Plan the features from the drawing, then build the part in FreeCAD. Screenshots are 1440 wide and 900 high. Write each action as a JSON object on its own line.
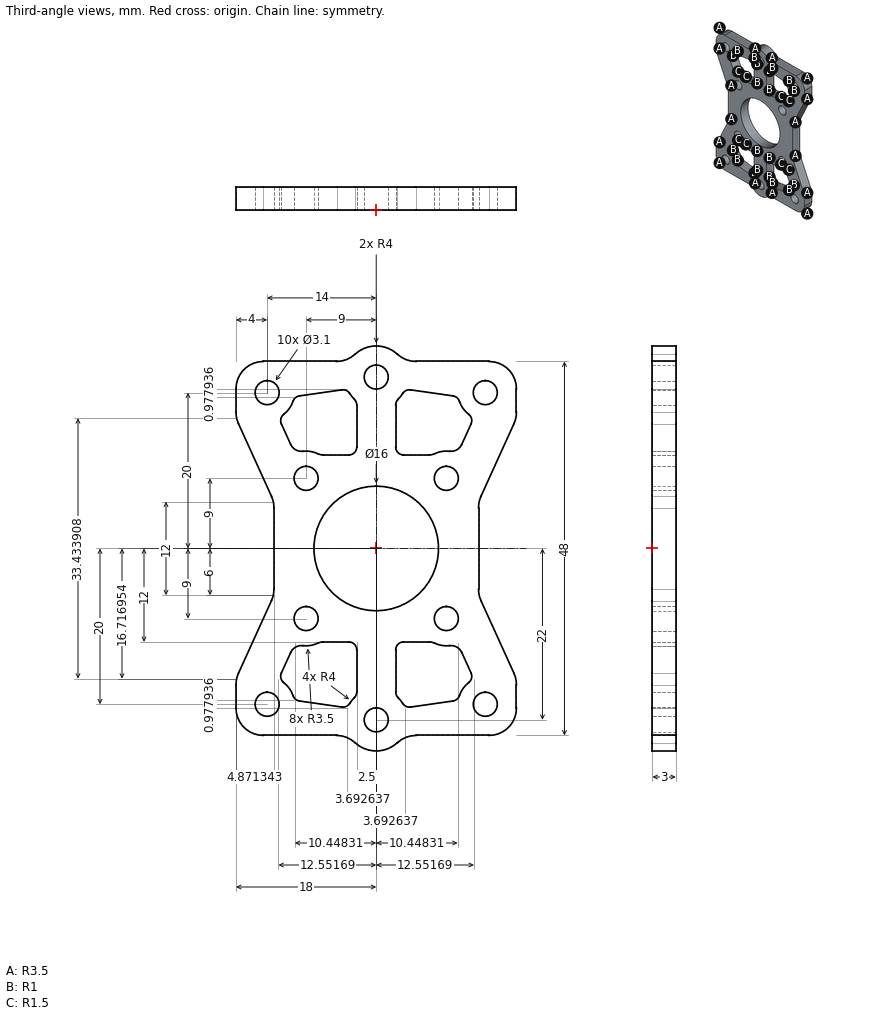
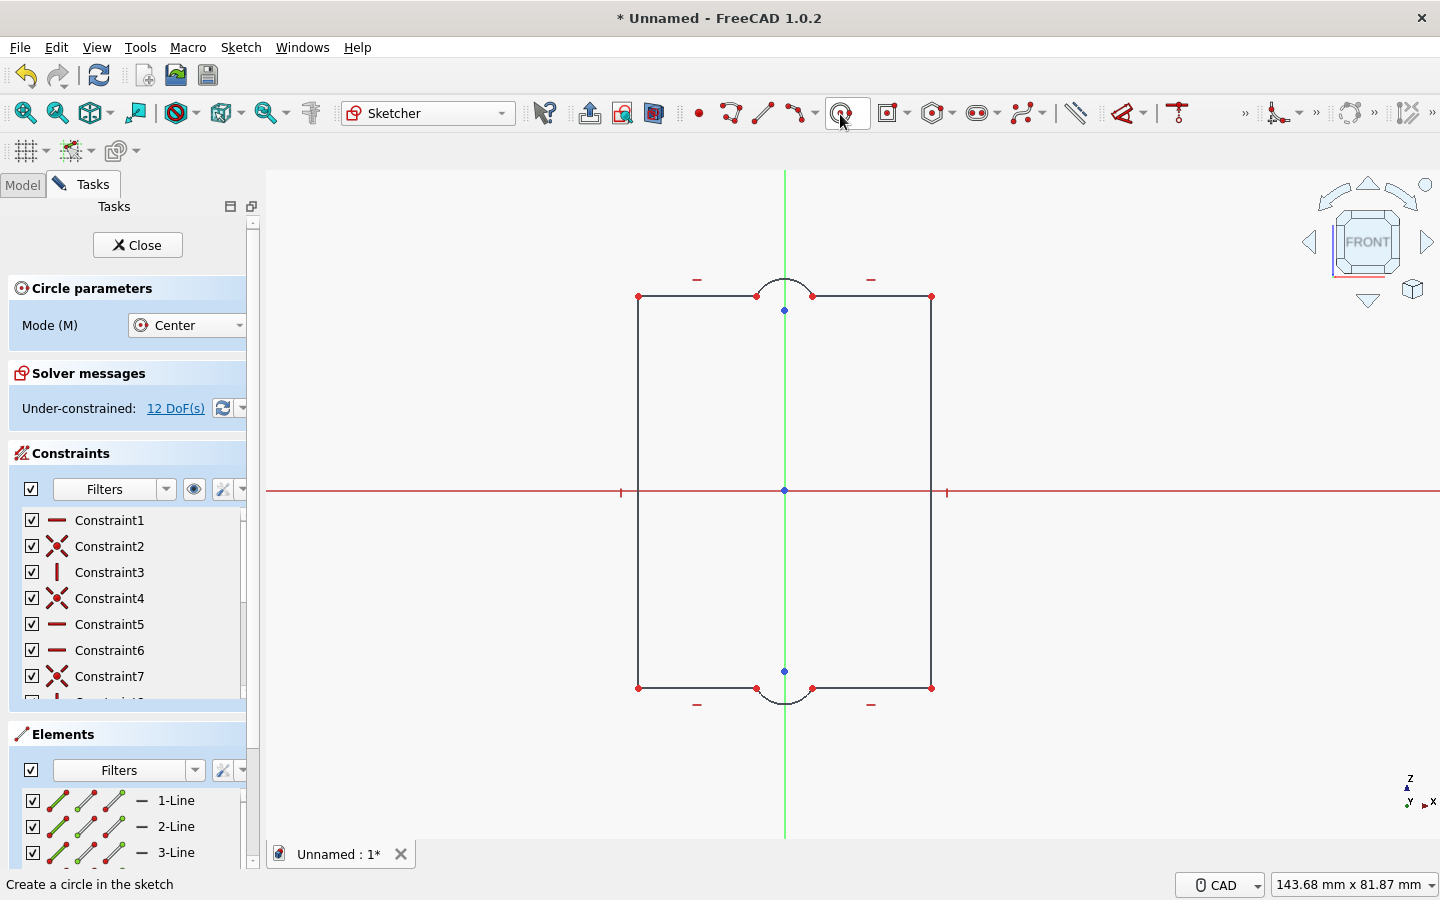
{"action": "scroll", "coordinate": [670, 327], "scroll_direction": "up", "scroll_amount": 3}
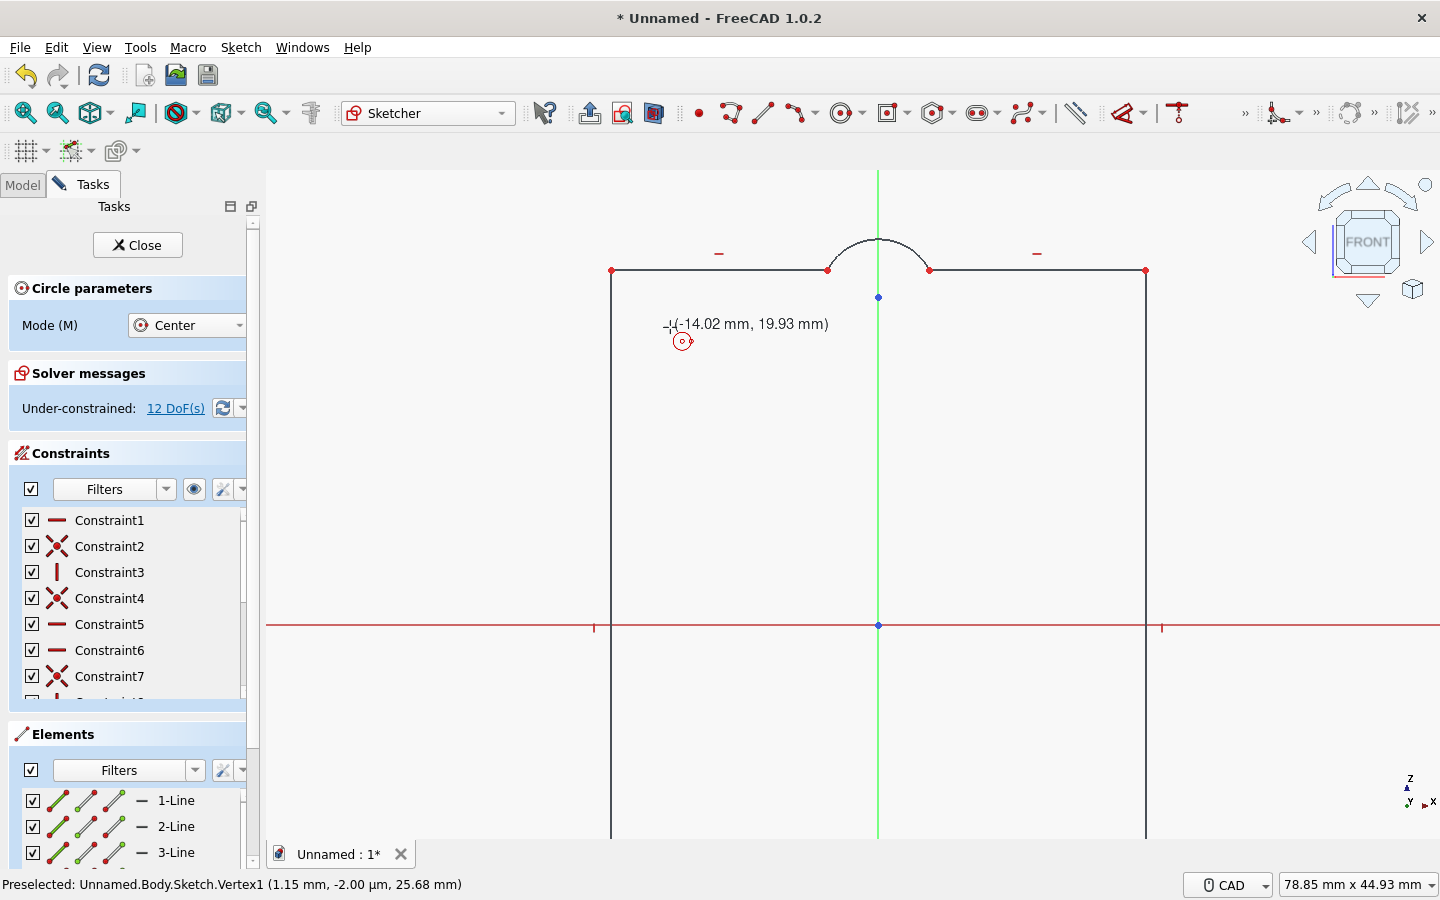
{"action": "left_click", "coordinate": [670, 328]}
{"action": "mouse_move", "coordinate": [686, 311]}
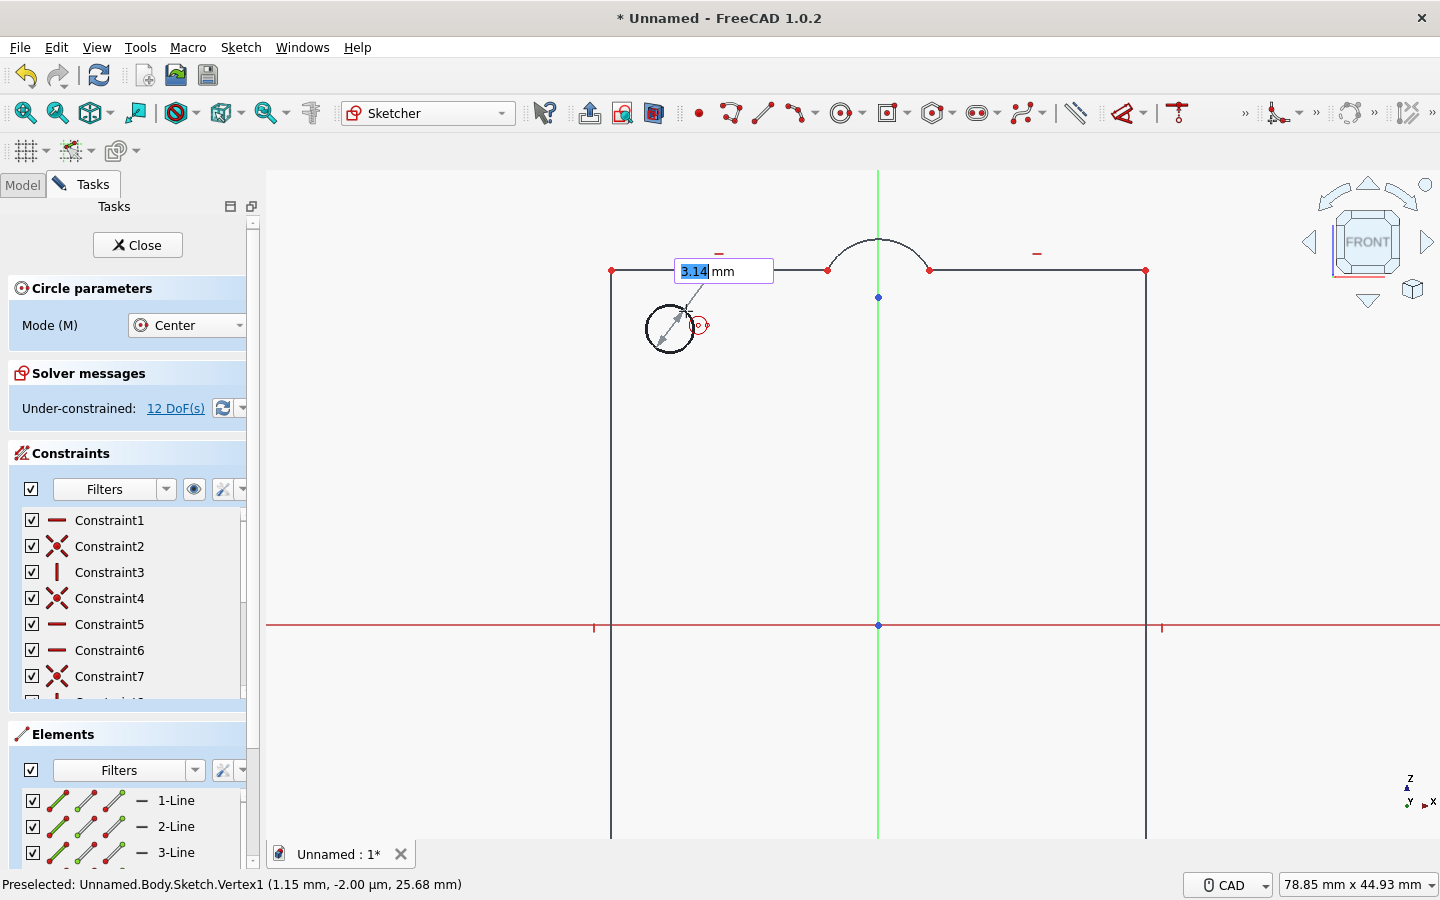
{"action": "type", "text": "3.1"}
{"action": "key", "text": "Return"}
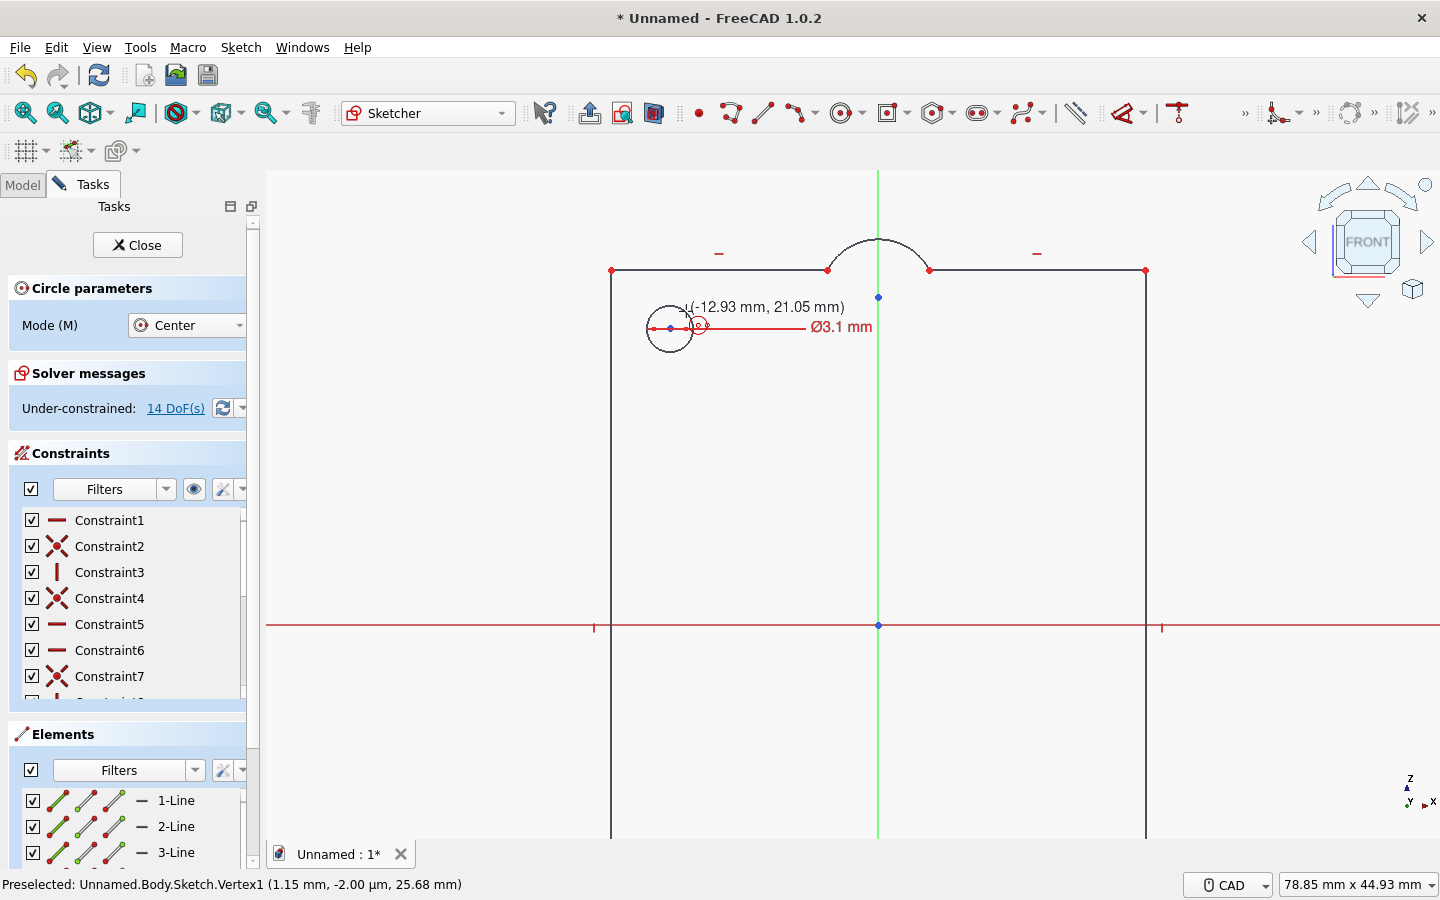
{"action": "left_click", "coordinate": [744, 491]}
{"action": "mouse_move", "coordinate": [761, 475]}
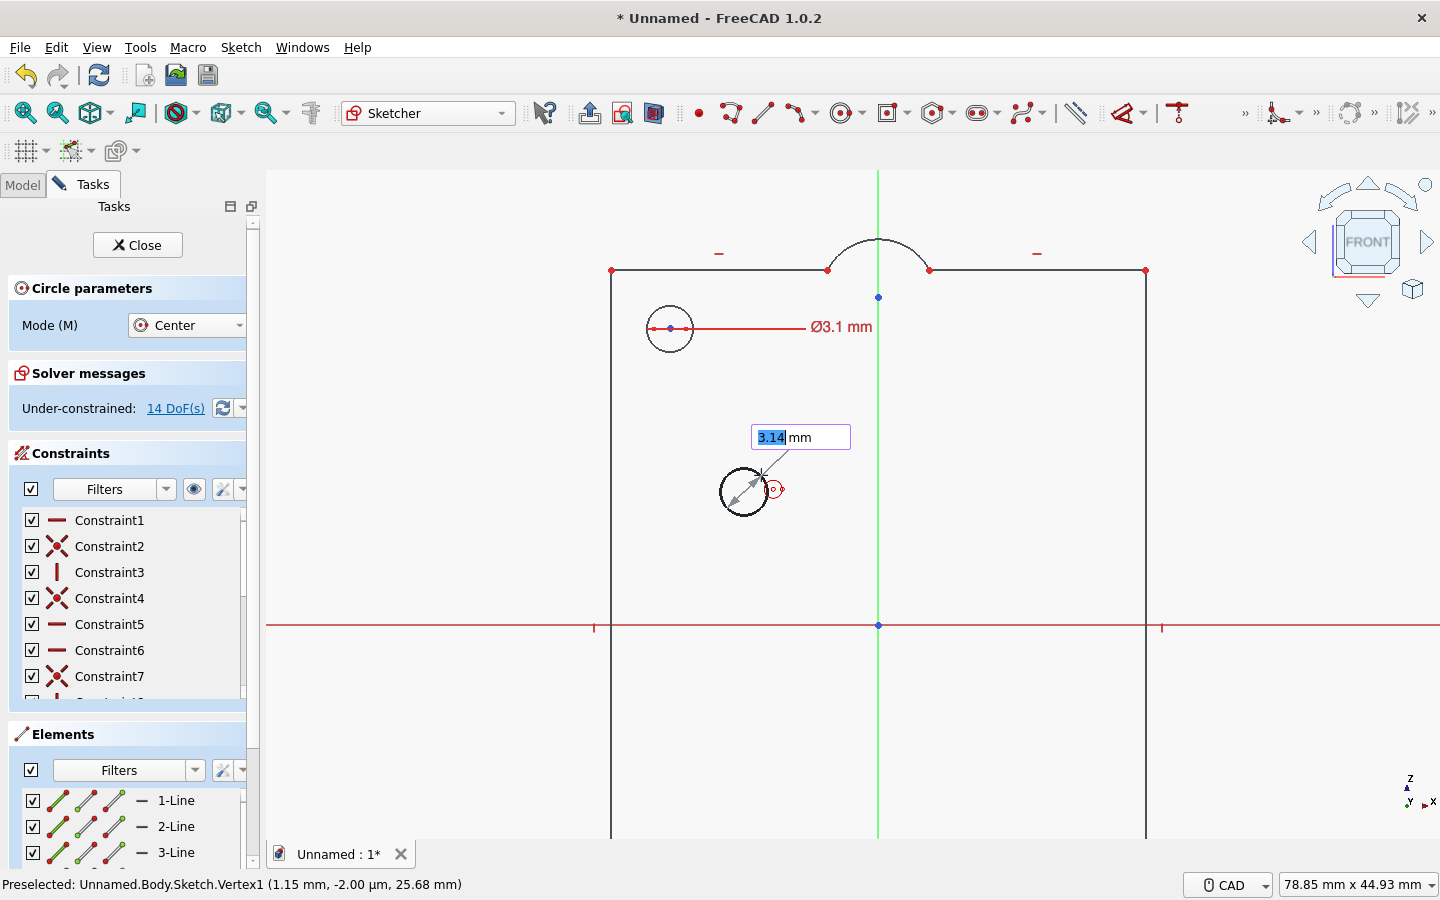
{"action": "type", "text": "3.1"}
{"action": "key", "text": "Return"}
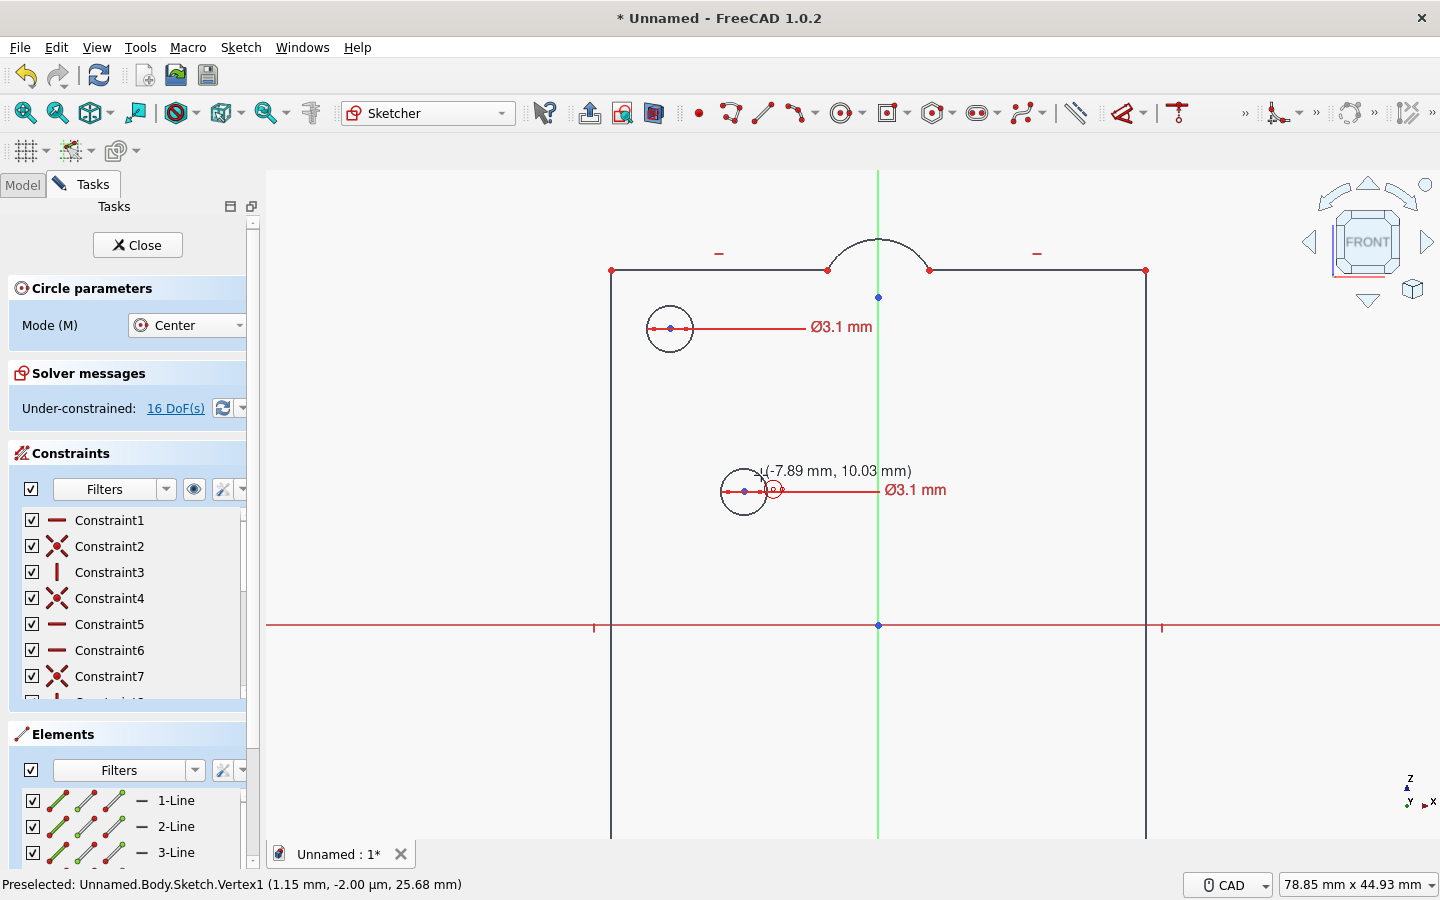
{"action": "left_click", "coordinate": [1087, 328]}
{"action": "mouse_move", "coordinate": [1103, 311]}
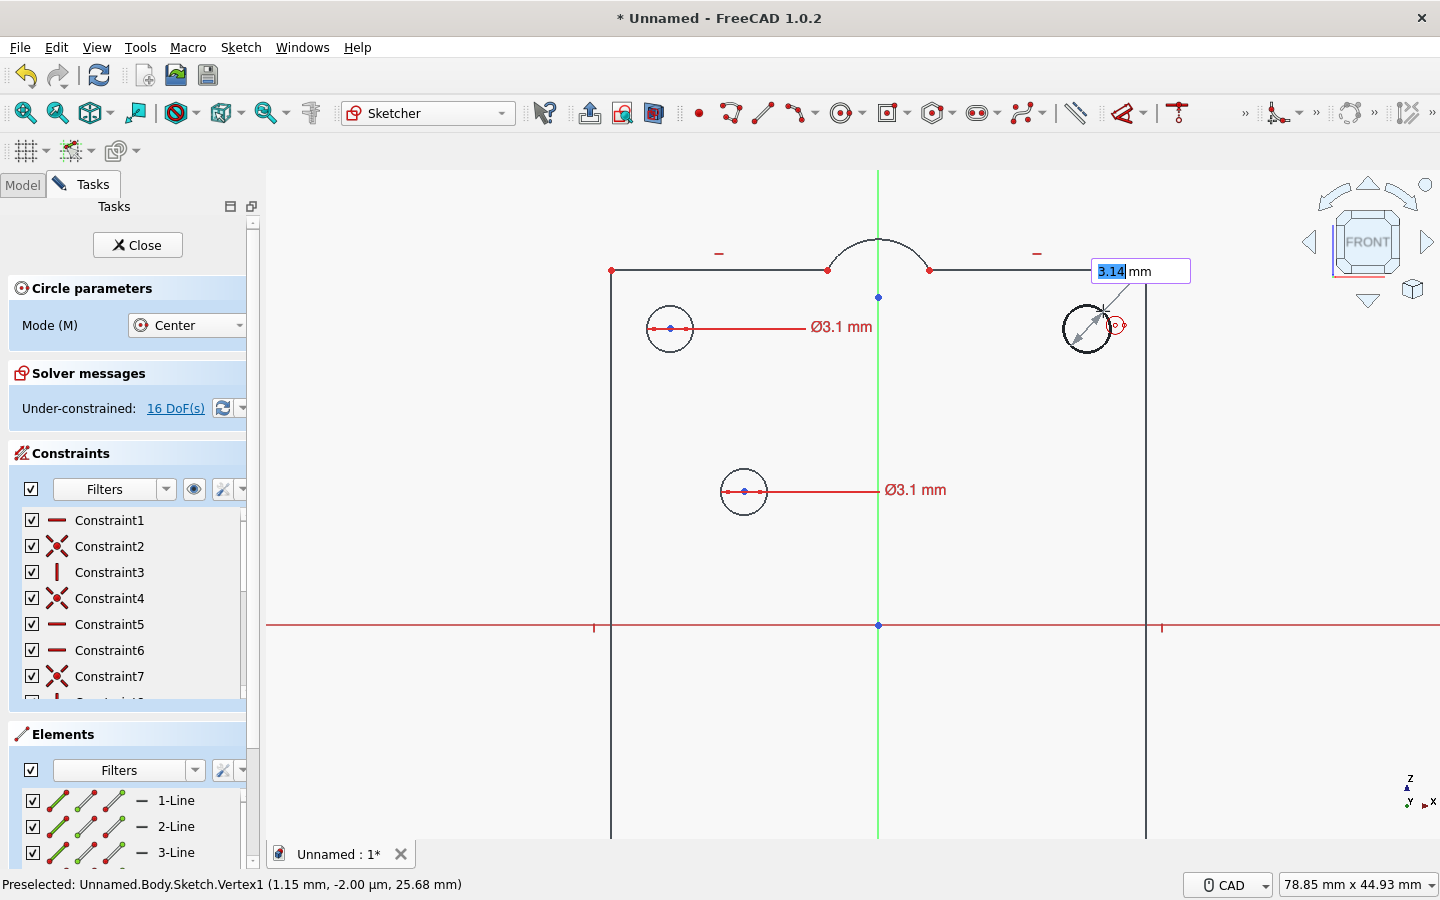
{"action": "type", "text": "3.1"}
{"action": "key", "text": "Return"}